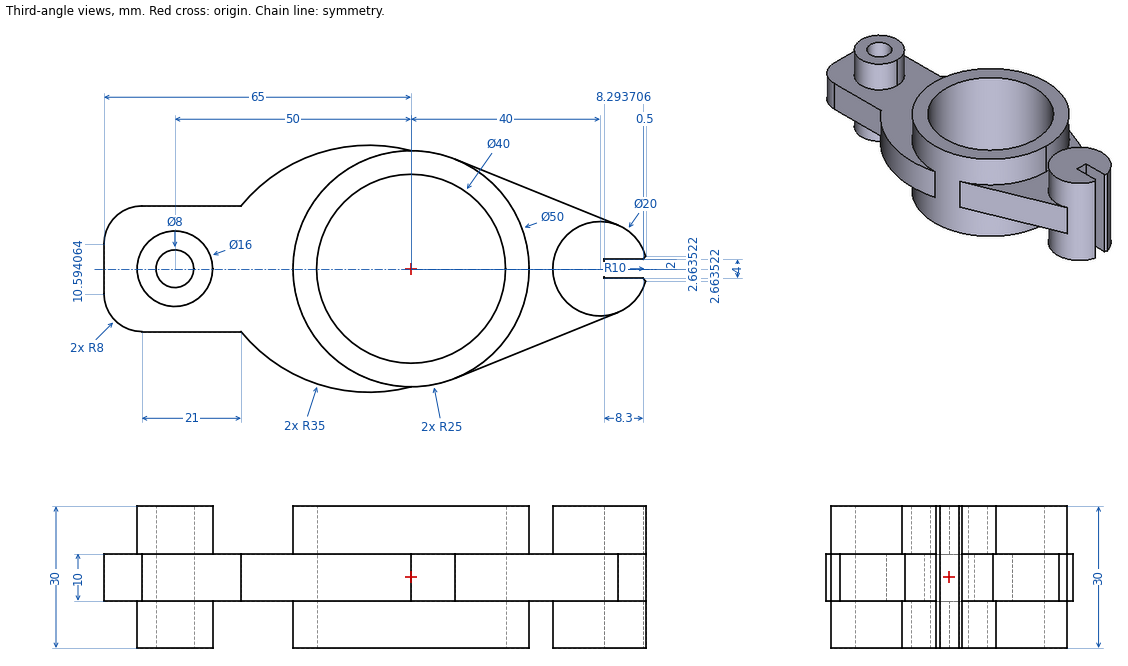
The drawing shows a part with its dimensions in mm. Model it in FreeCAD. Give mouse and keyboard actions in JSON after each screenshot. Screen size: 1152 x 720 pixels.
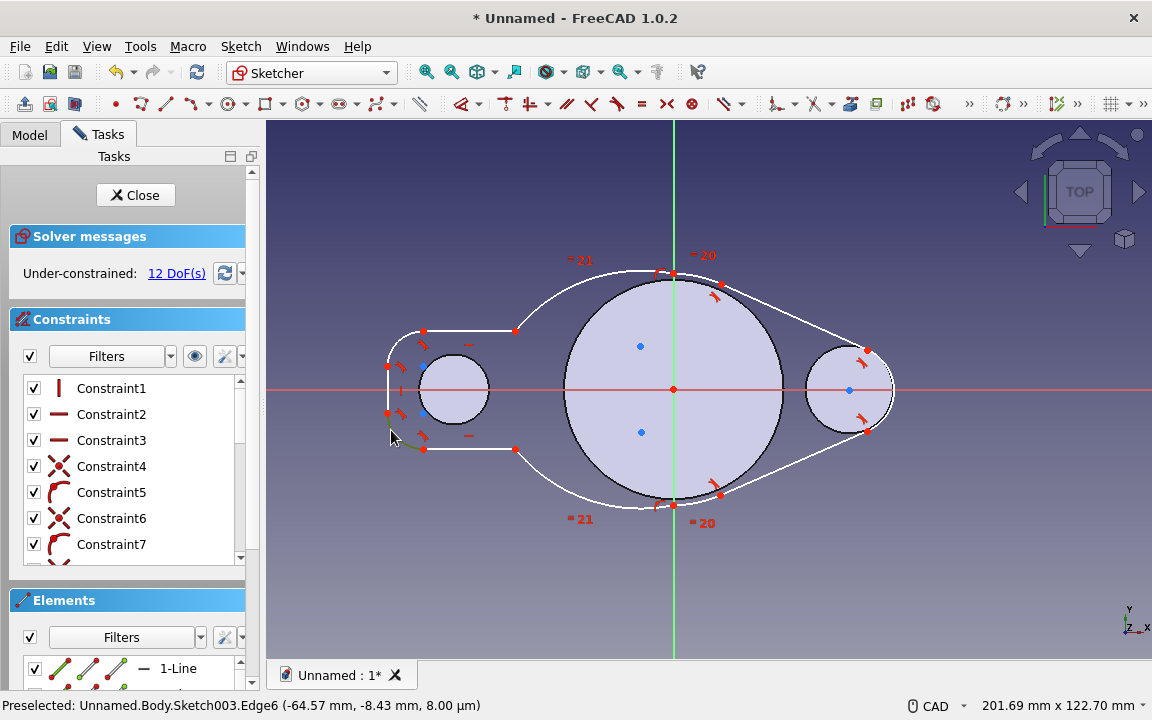
{"action": "left_click", "coordinate": [407, 335]}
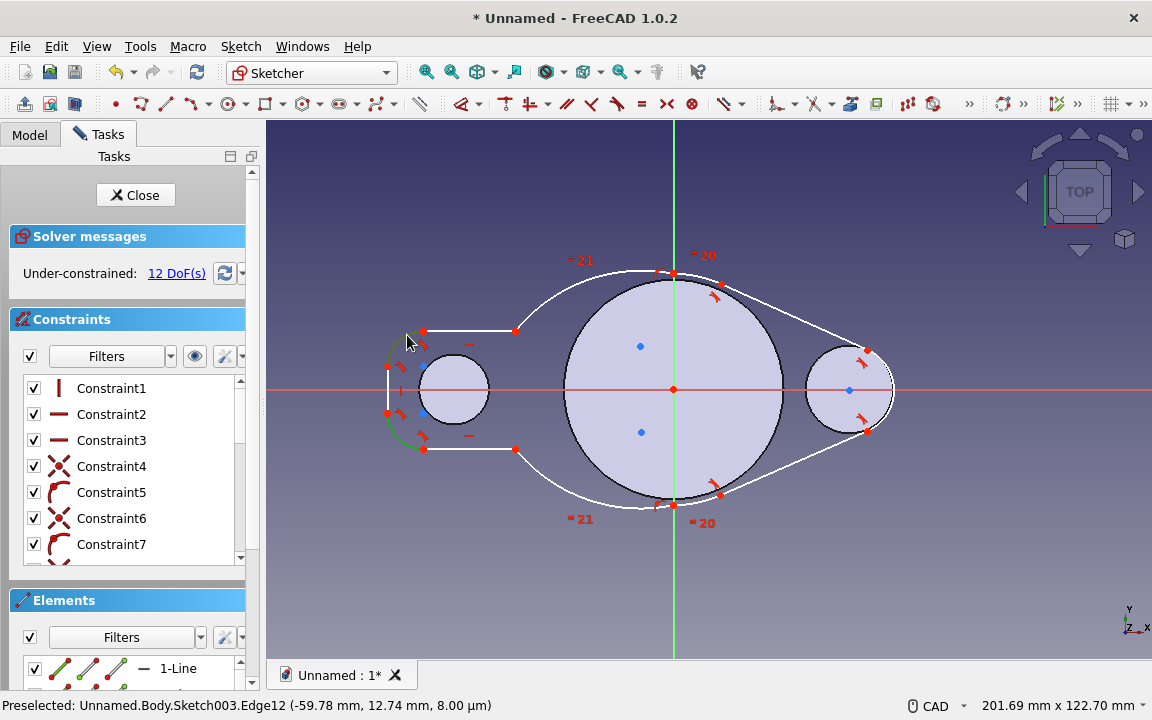
{"action": "key", "text": "e"}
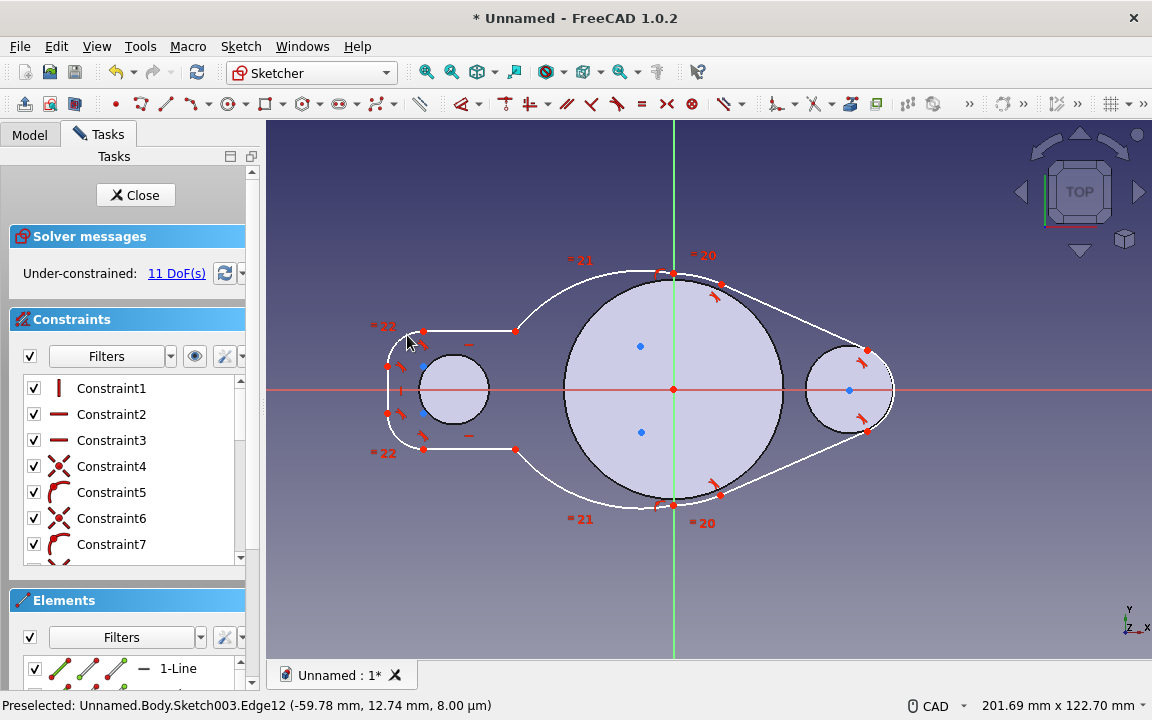
{"action": "left_click", "coordinate": [850, 390]}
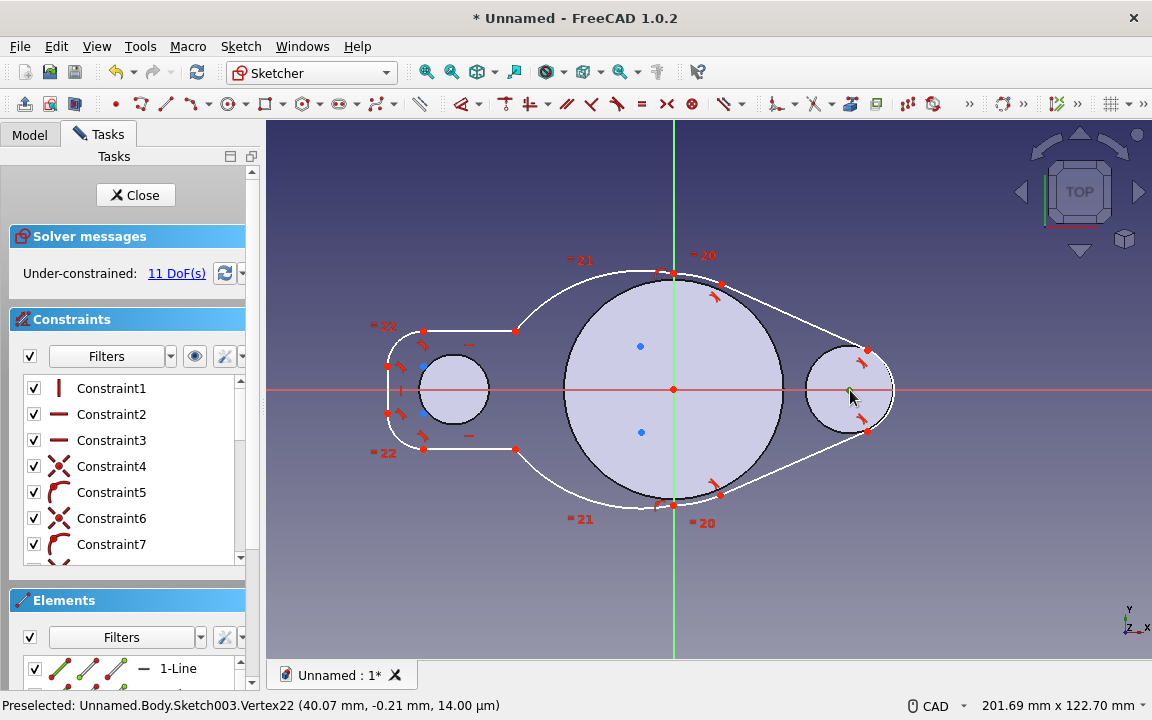
{"action": "left_click", "coordinate": [344, 390]}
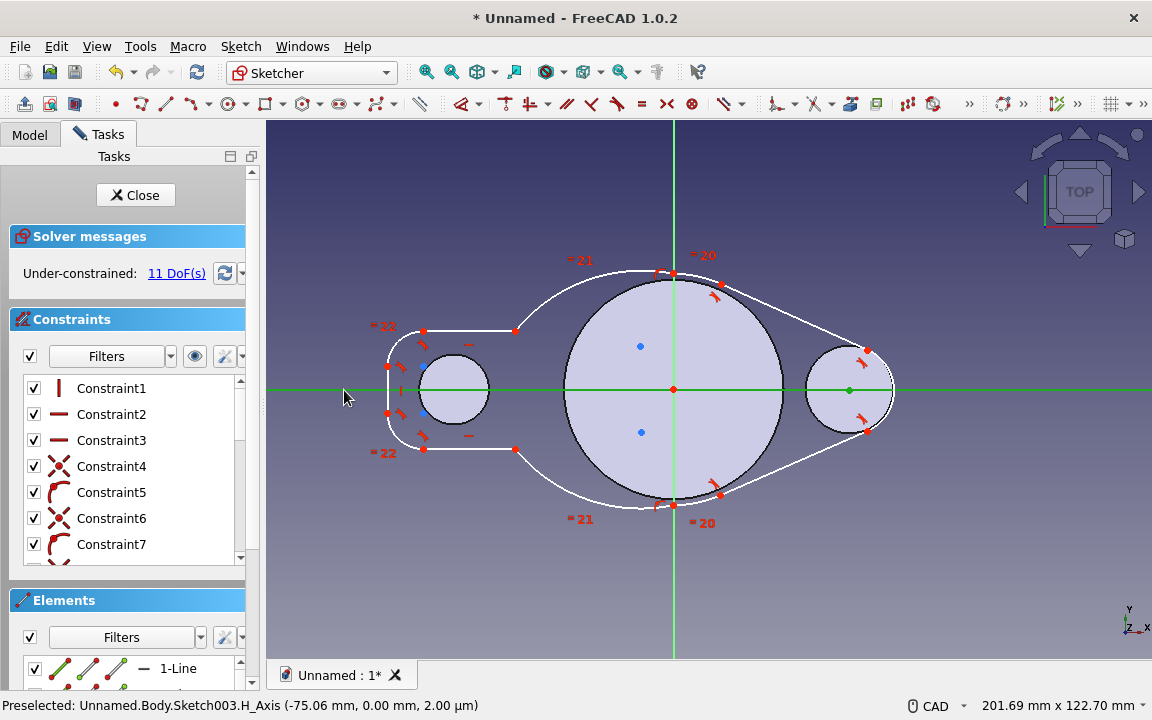
{"action": "left_click", "coordinate": [505, 104]}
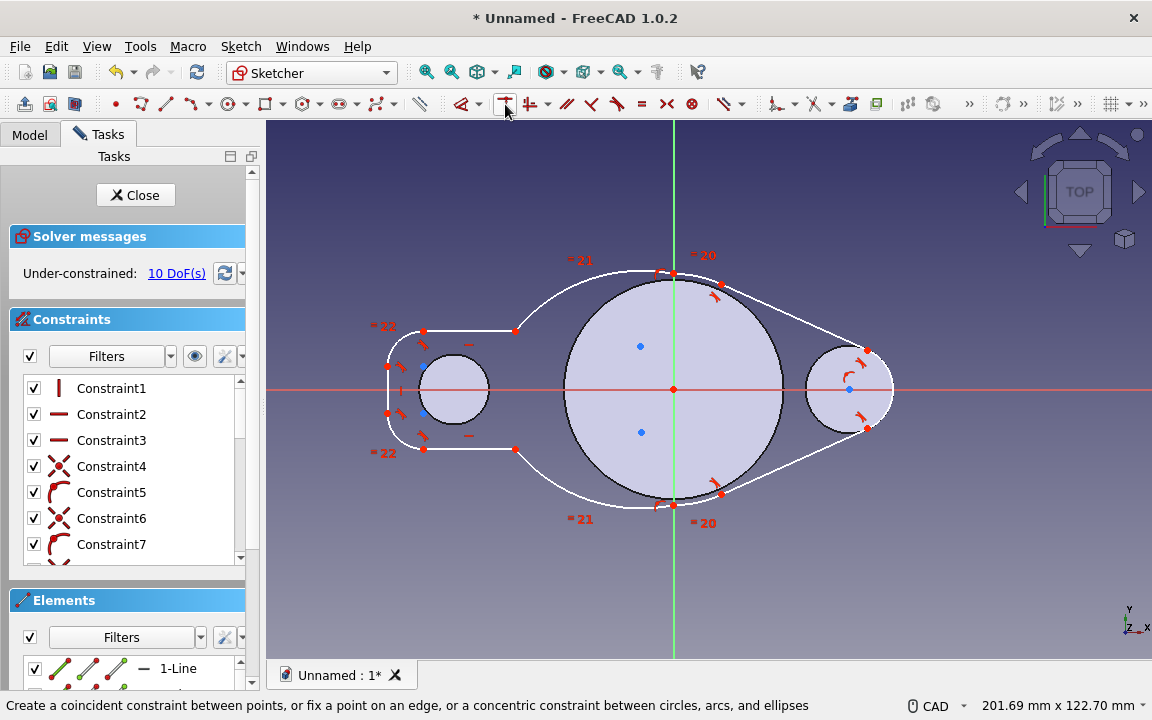
{"action": "left_click", "coordinate": [515, 449]}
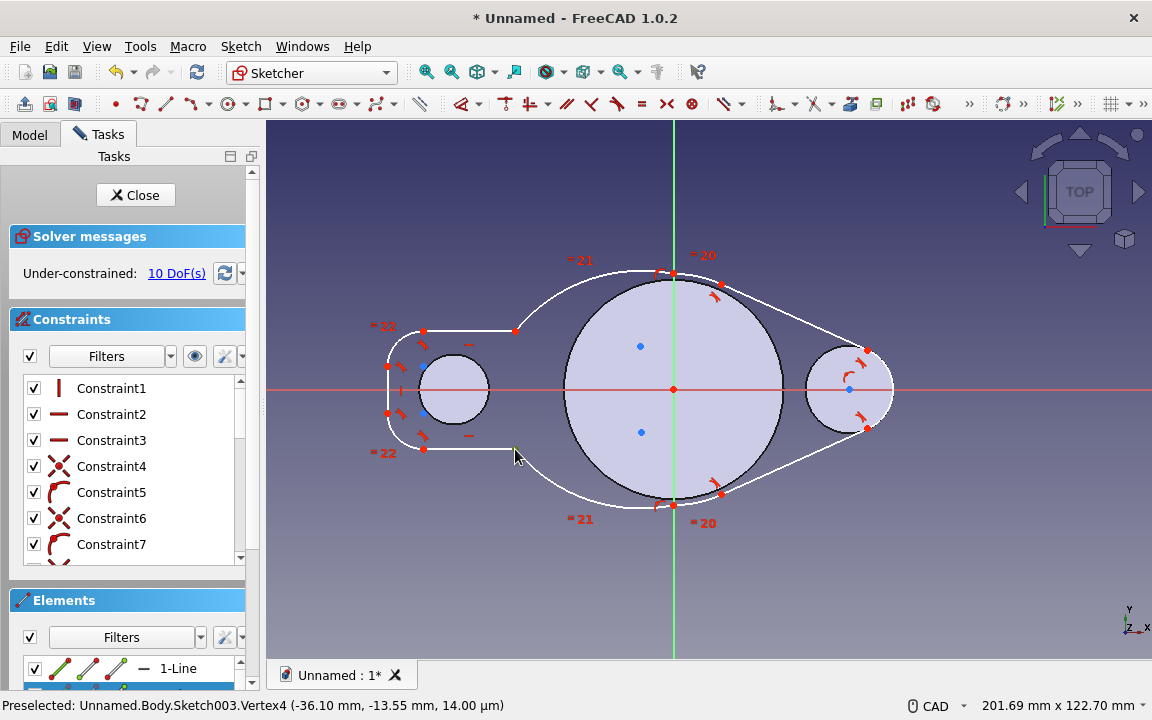
{"action": "left_click", "coordinate": [515, 331]}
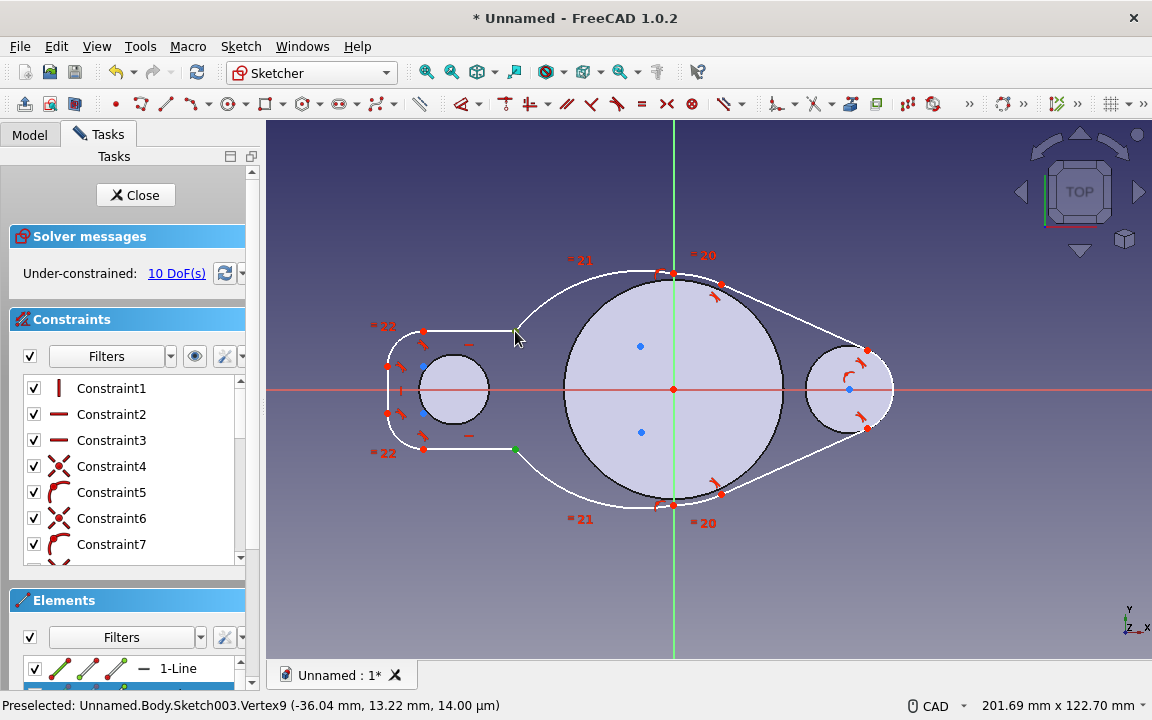
{"action": "left_click", "coordinate": [344, 390]}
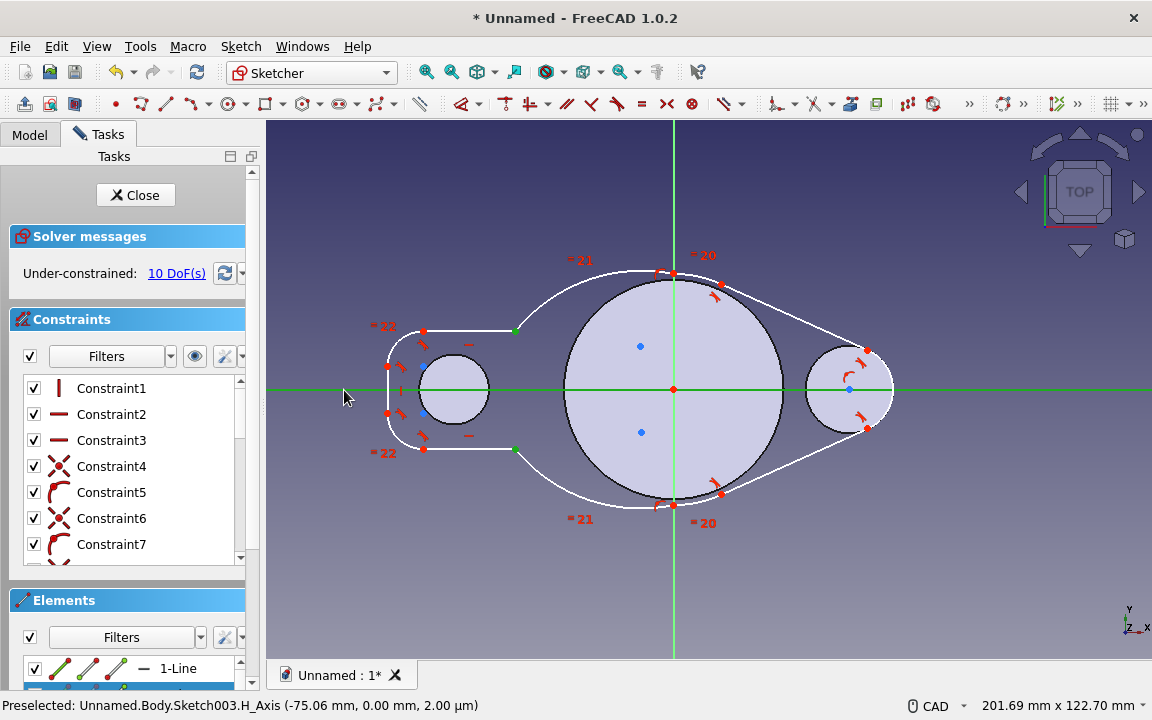
{"action": "left_click", "coordinate": [667, 104]}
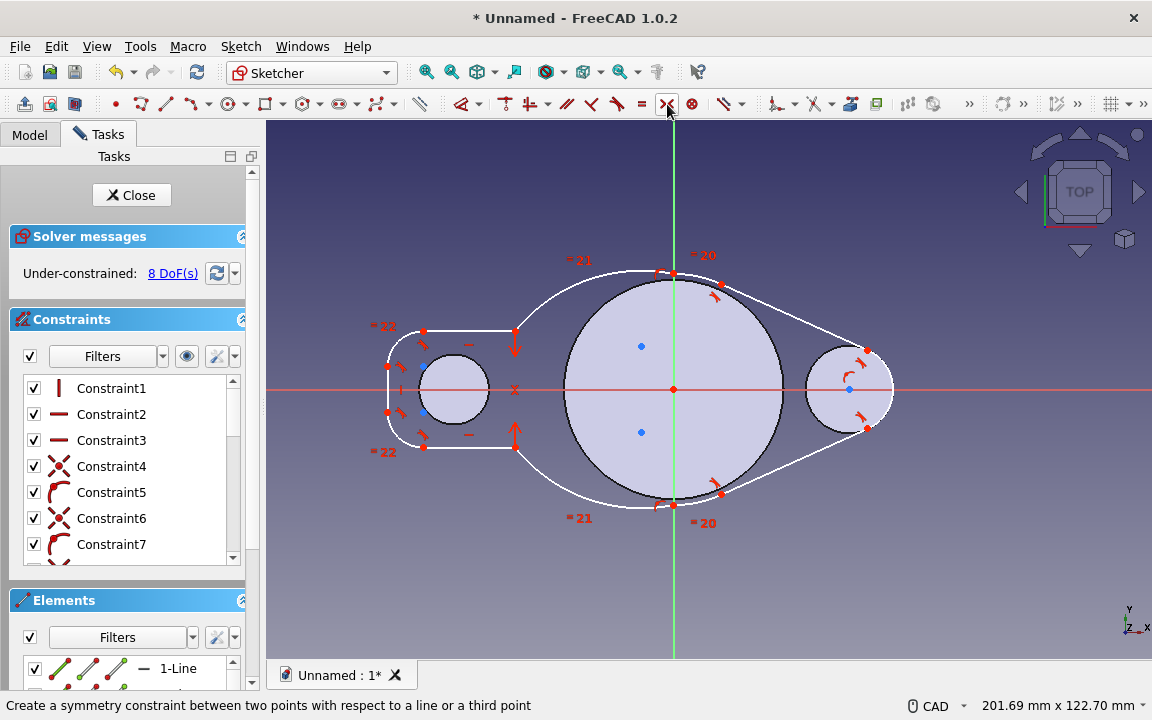
{"action": "left_click", "coordinate": [460, 104]}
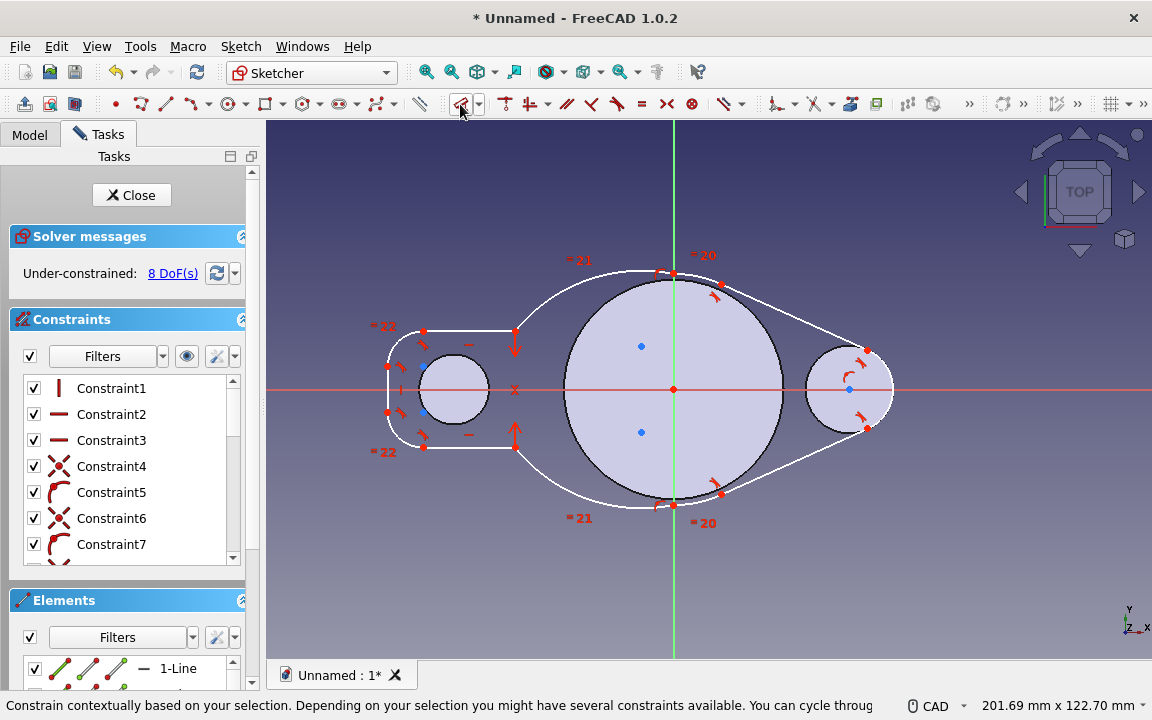
{"action": "left_click", "coordinate": [392, 428]}
{"action": "left_click", "coordinate": [363, 443]}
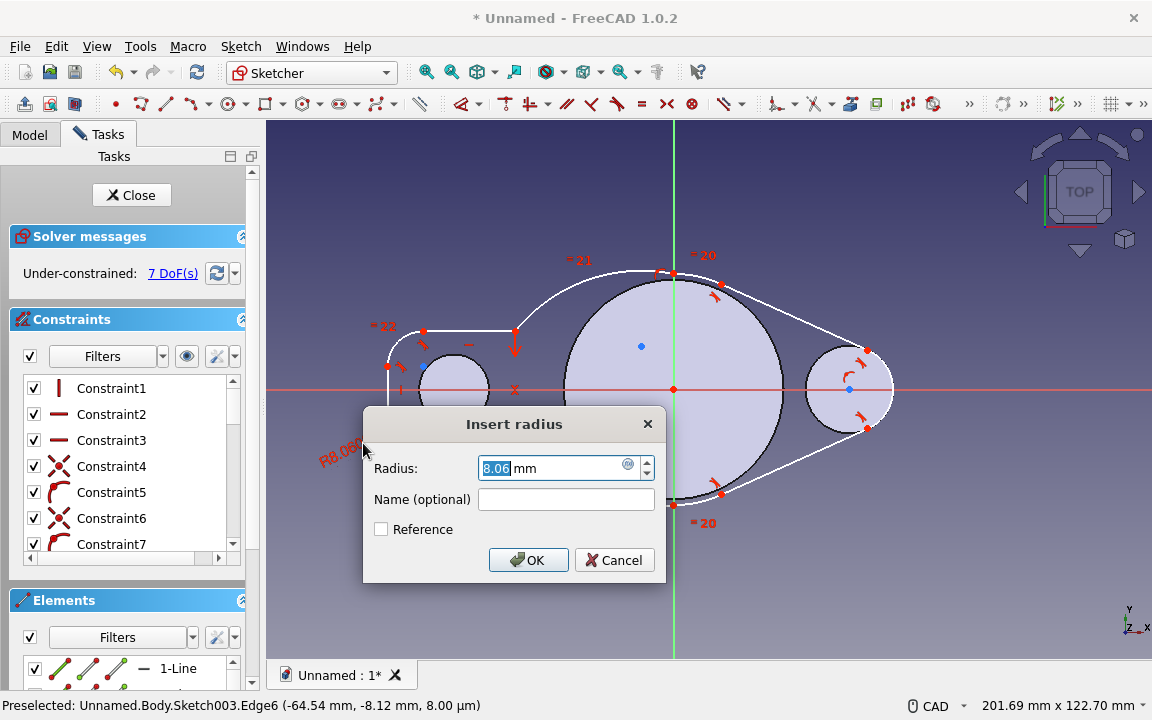
{"action": "type", "text": "8"}
{"action": "key", "text": "Return"}